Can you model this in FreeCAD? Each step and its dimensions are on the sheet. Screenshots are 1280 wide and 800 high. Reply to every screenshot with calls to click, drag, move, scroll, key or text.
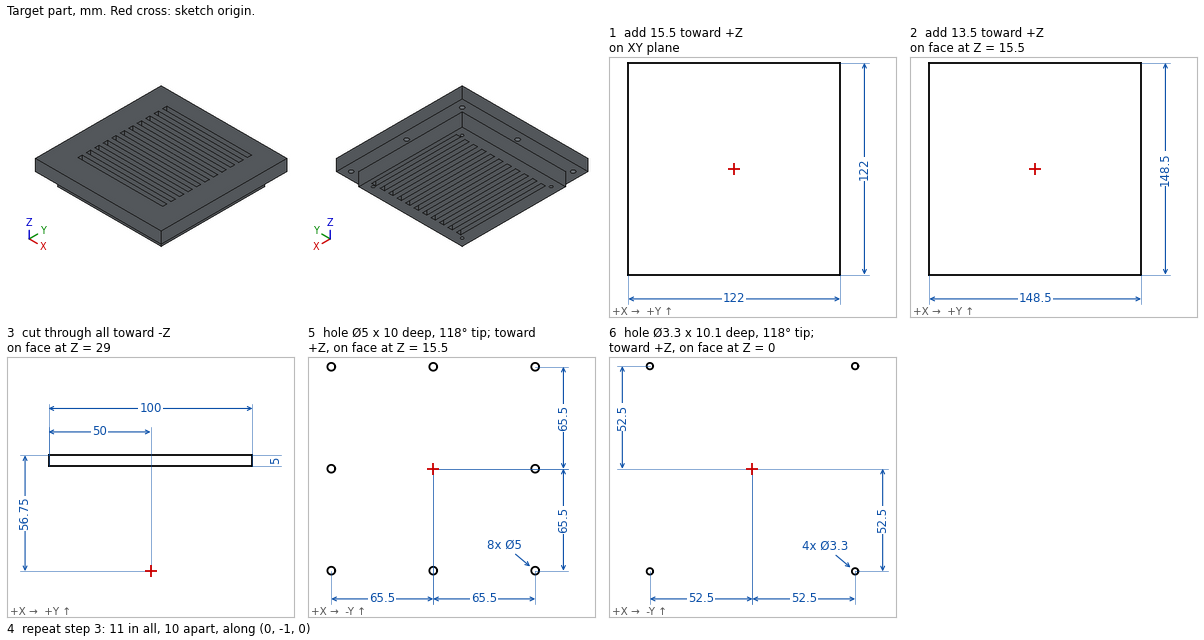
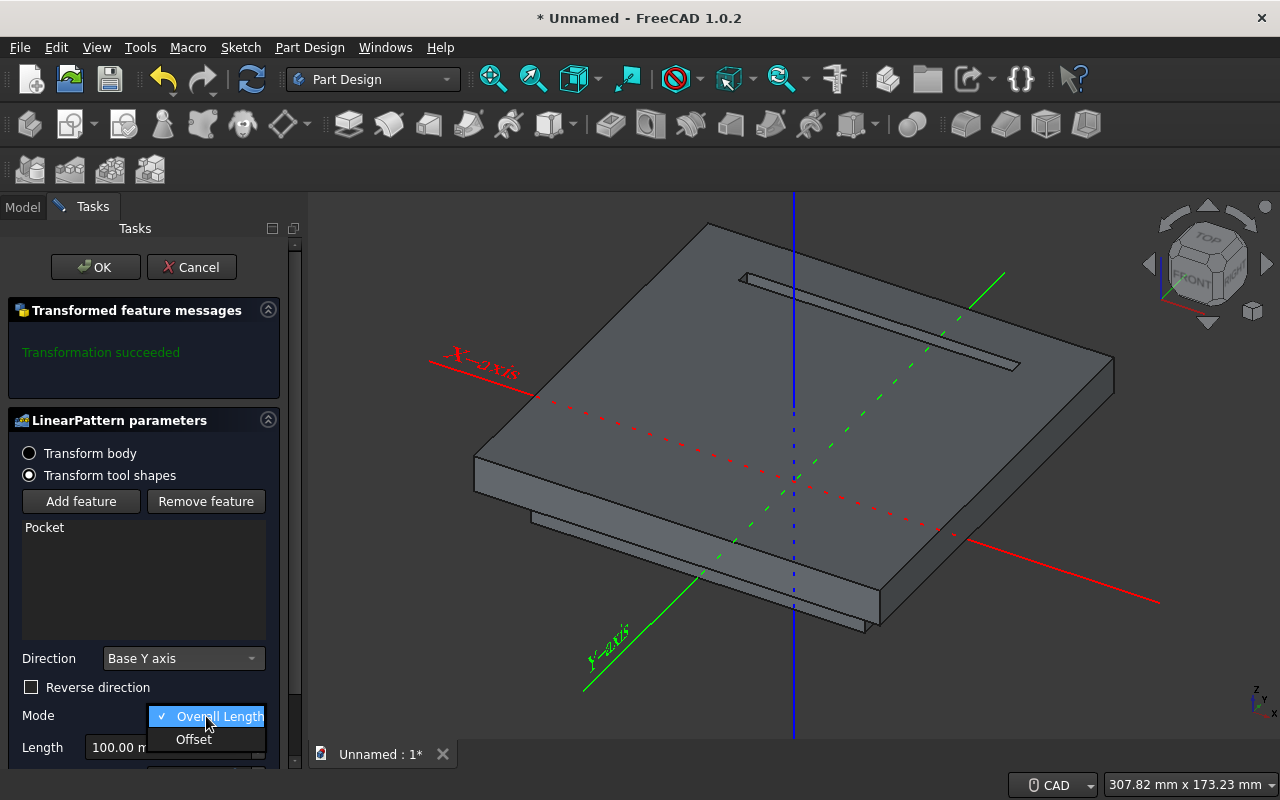
click(206, 740)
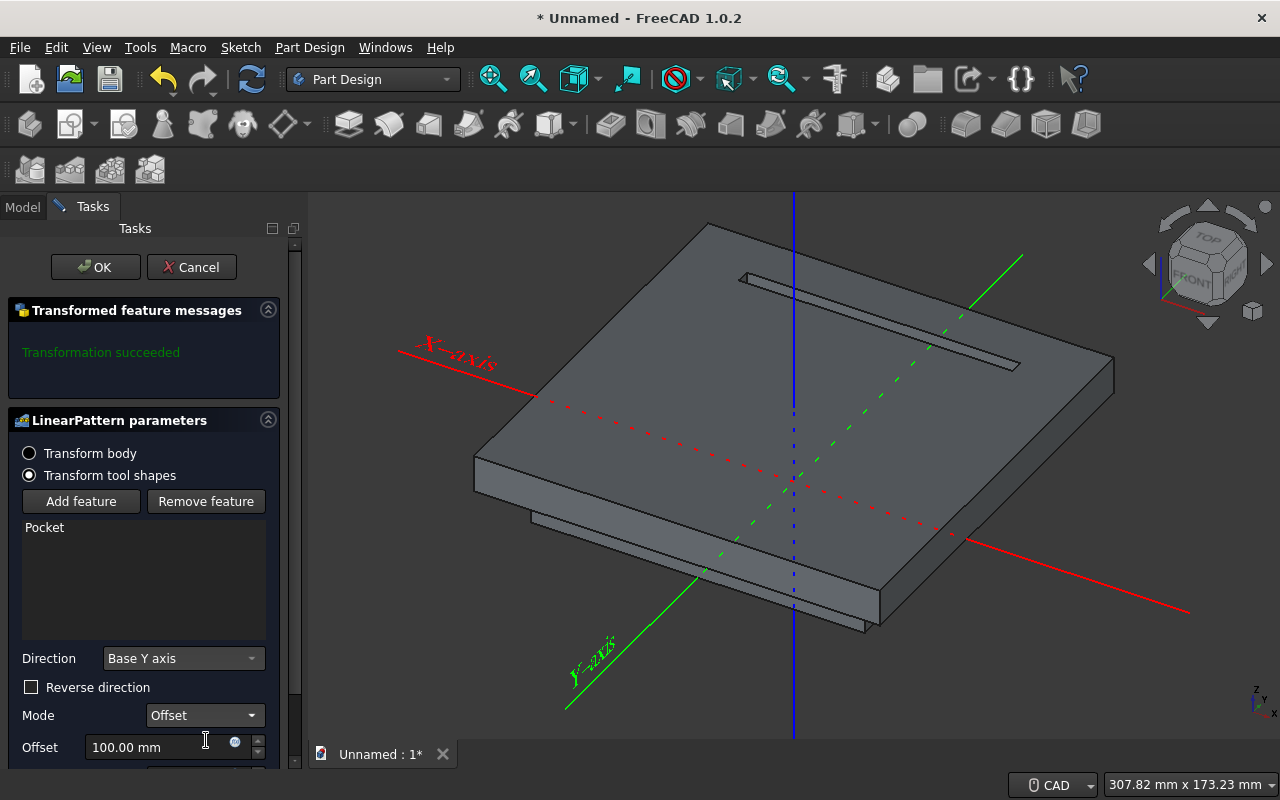
triple_click(168, 747)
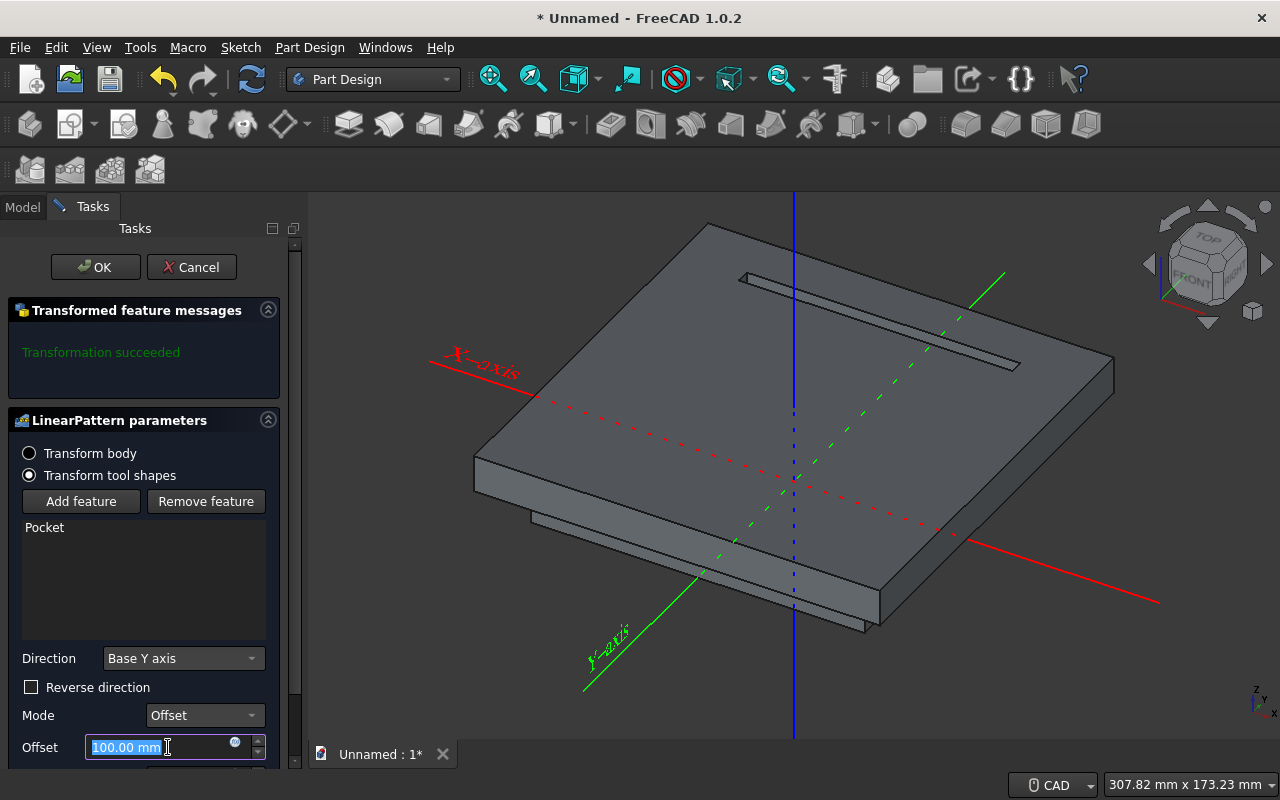
text(10)
key(Tab)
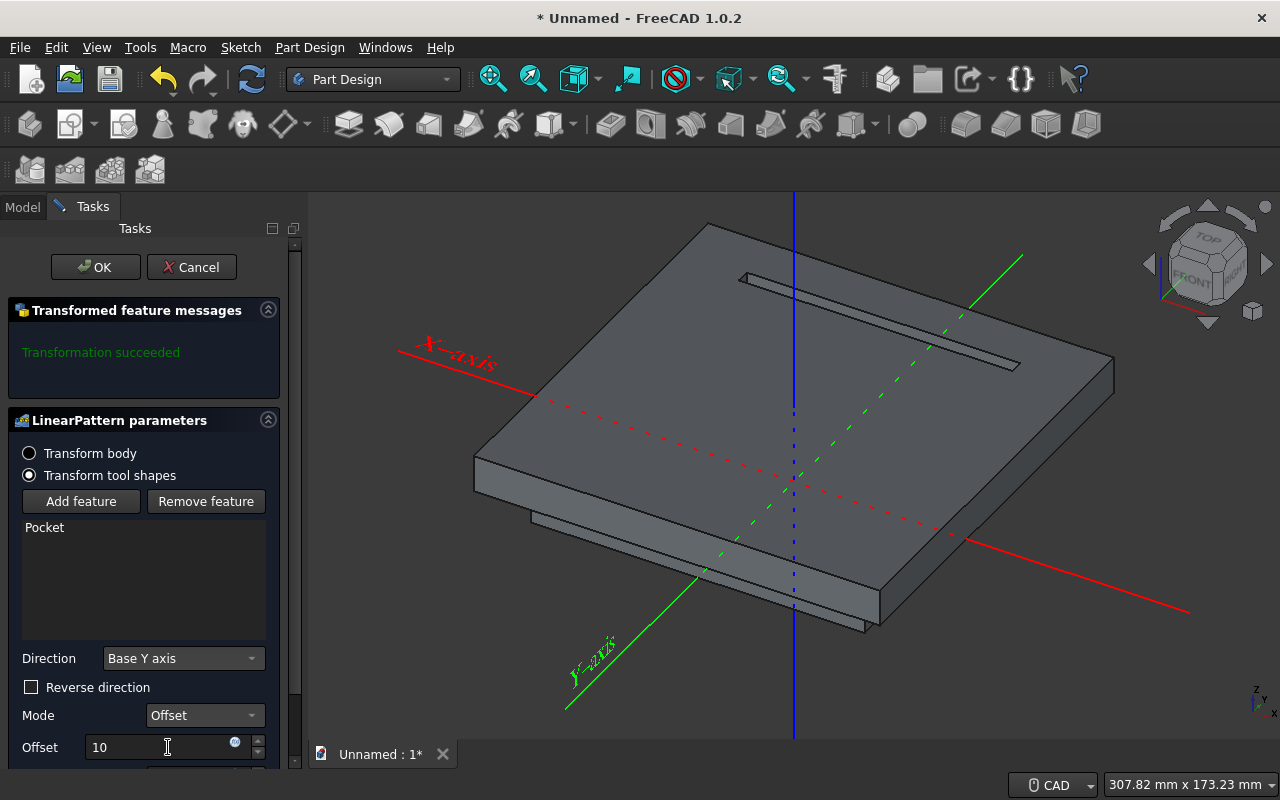
scroll(295, 503, down, 2)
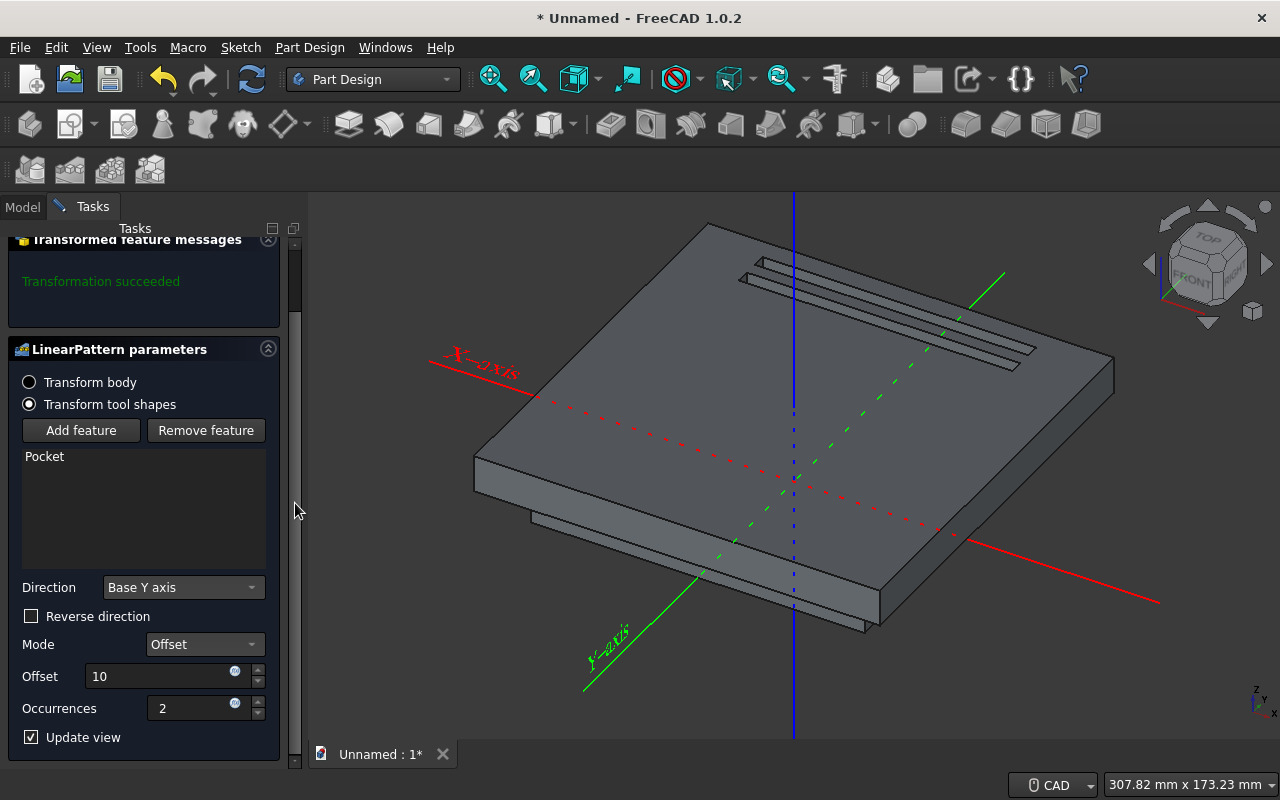
triple_click(198, 708)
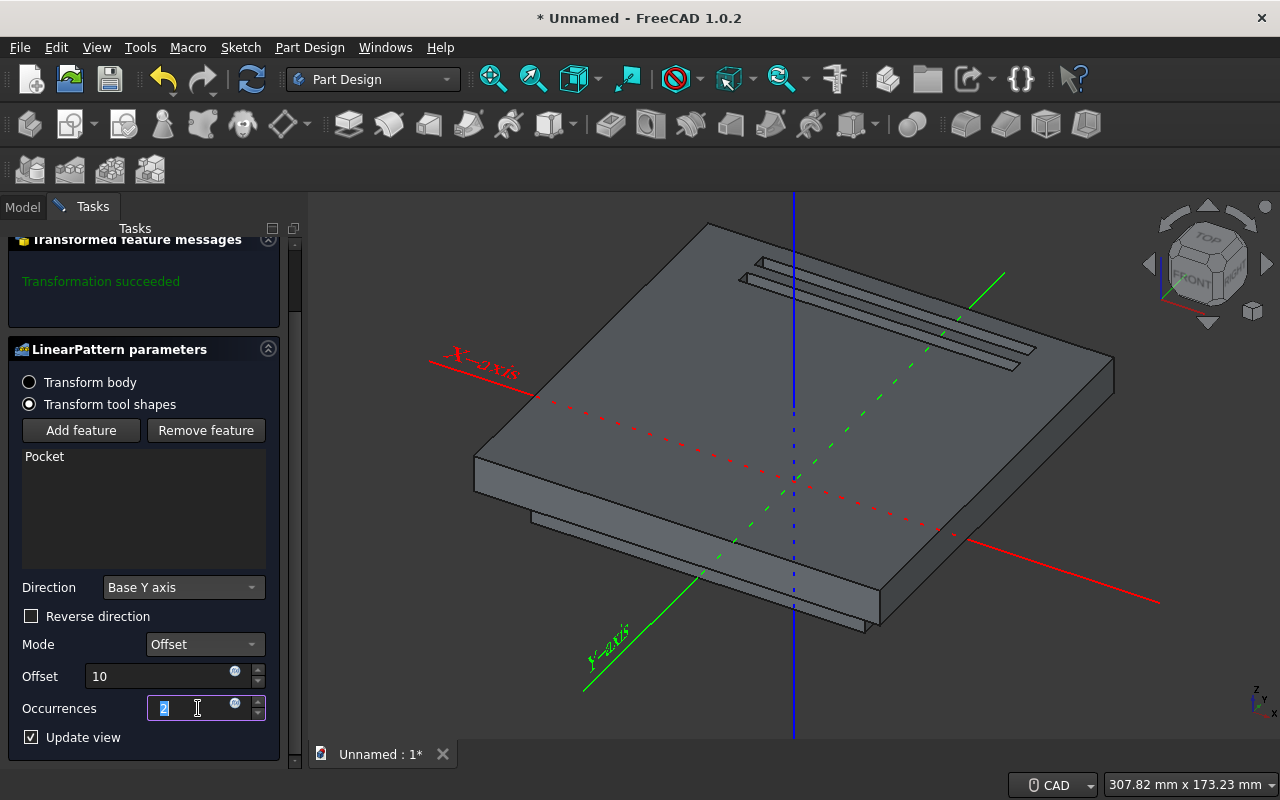
text(11)
key(Tab)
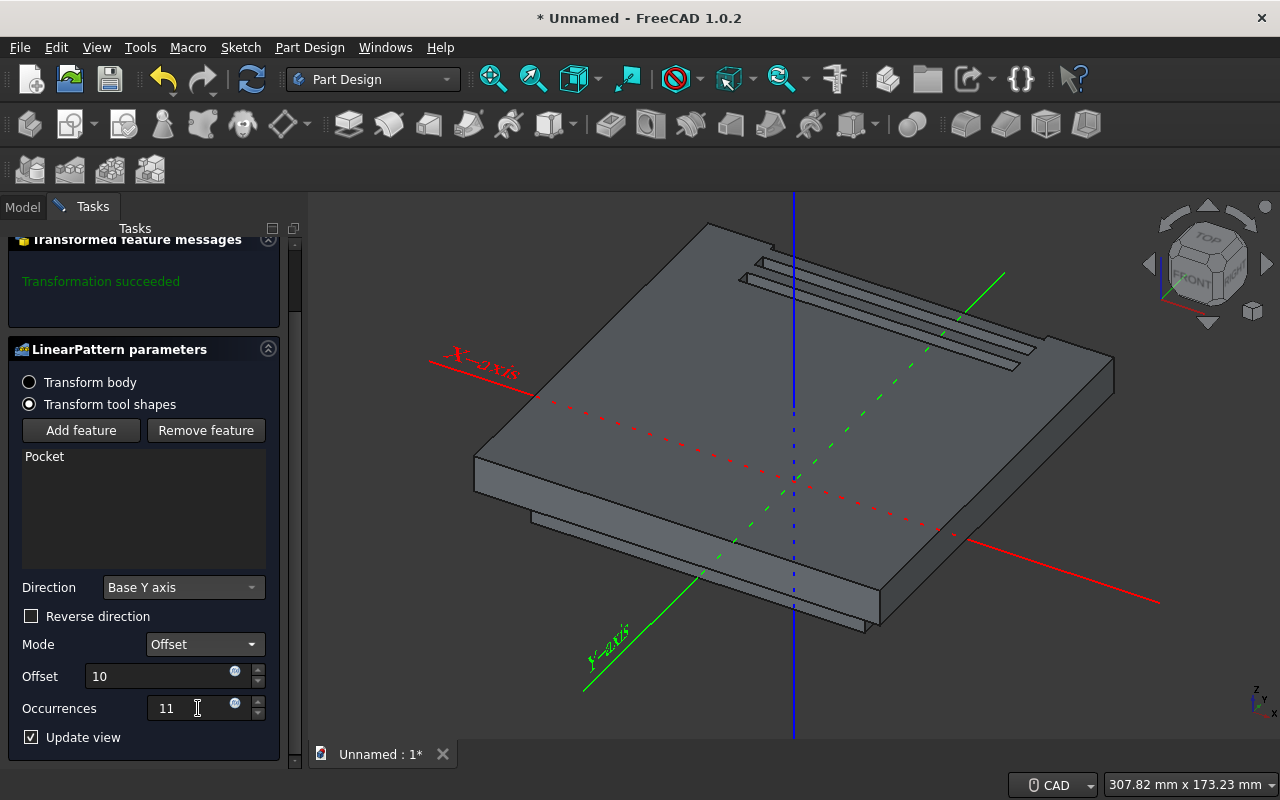
click(30, 616)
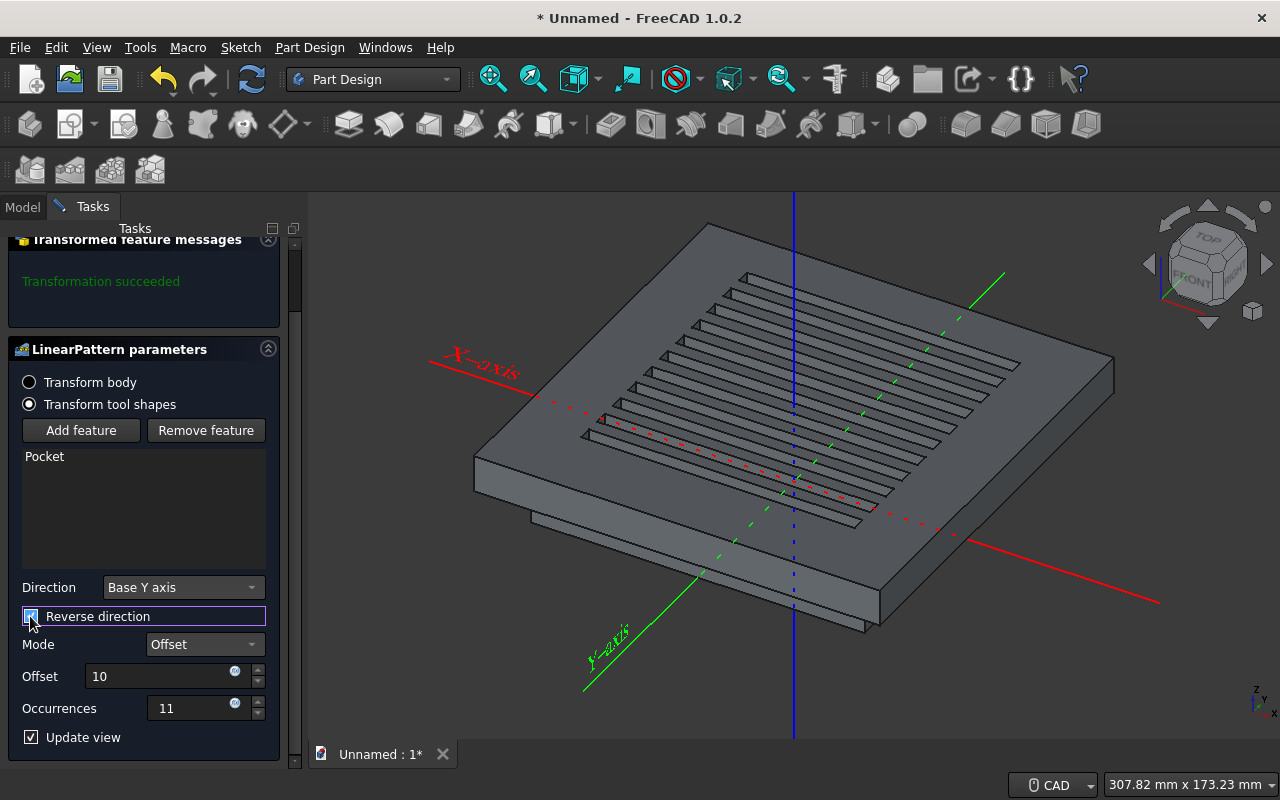
scroll(295, 503, up, 2)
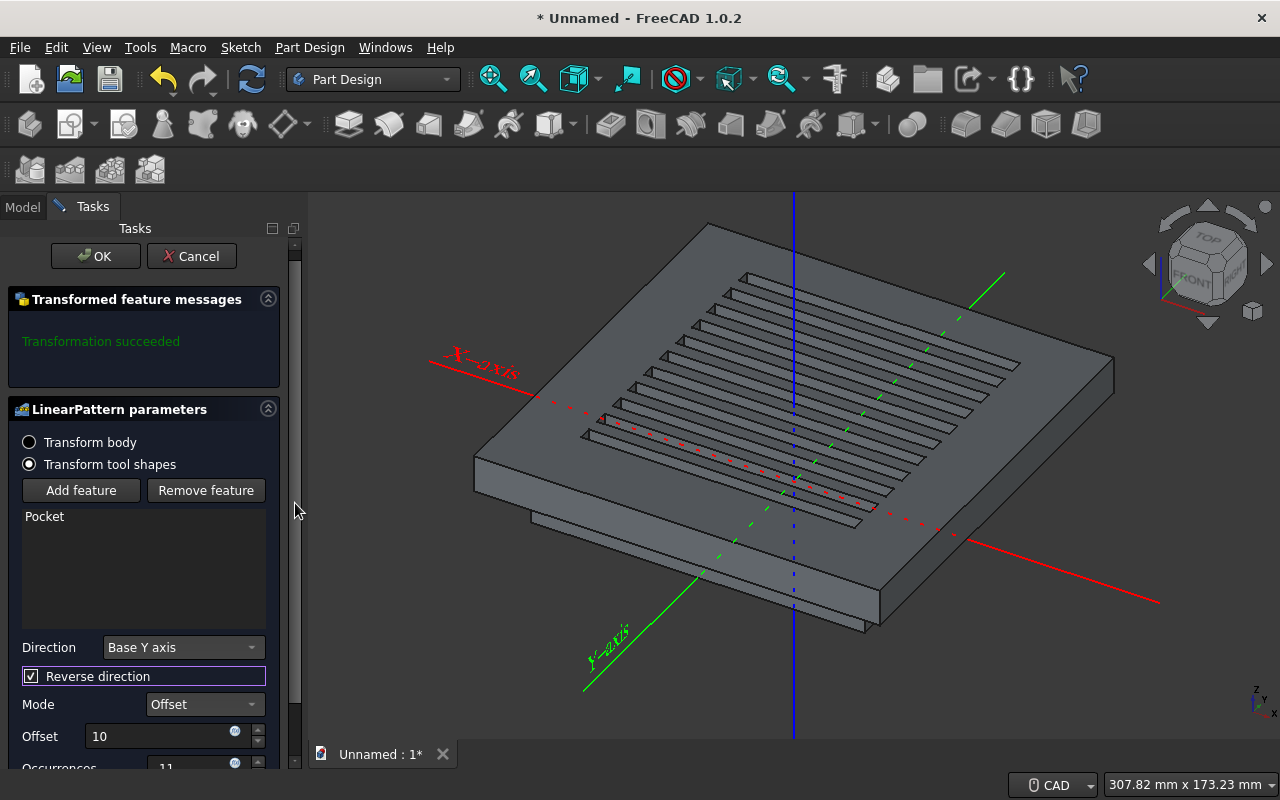
click(96, 267)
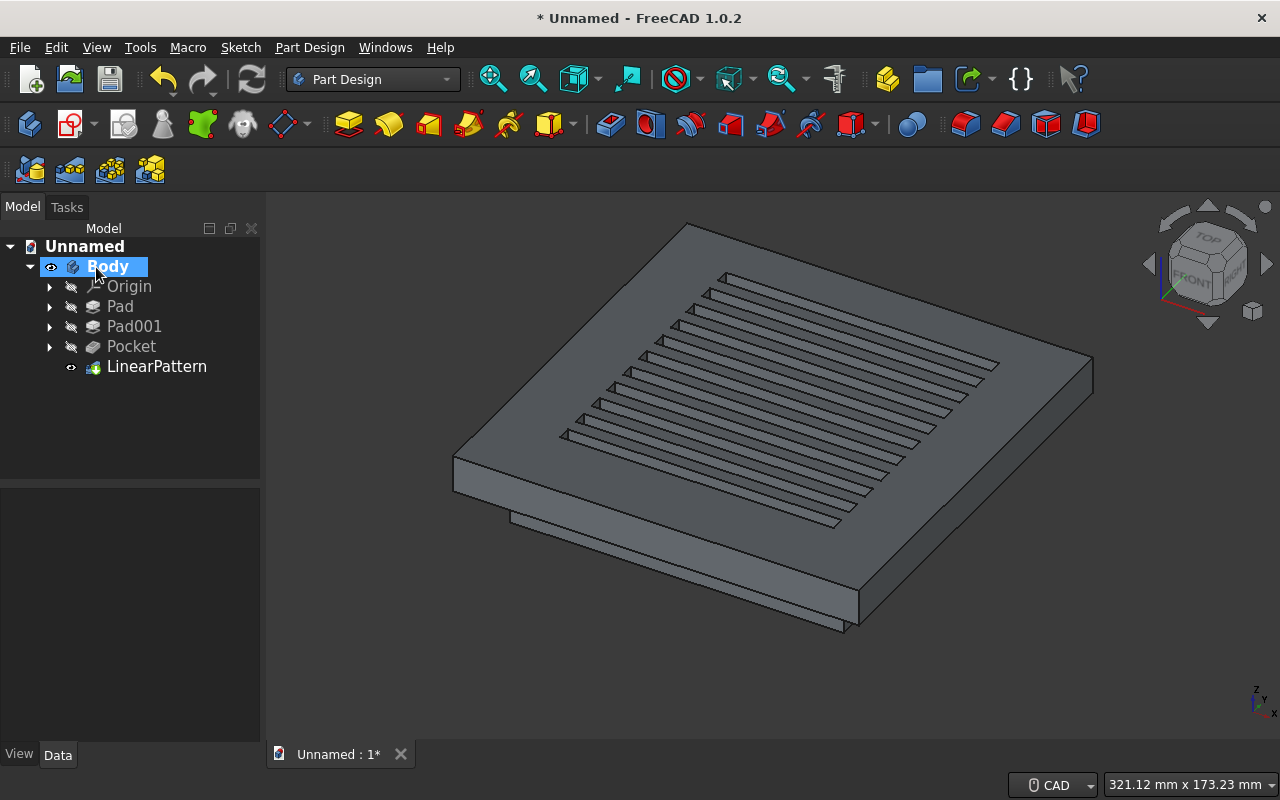
key(5)